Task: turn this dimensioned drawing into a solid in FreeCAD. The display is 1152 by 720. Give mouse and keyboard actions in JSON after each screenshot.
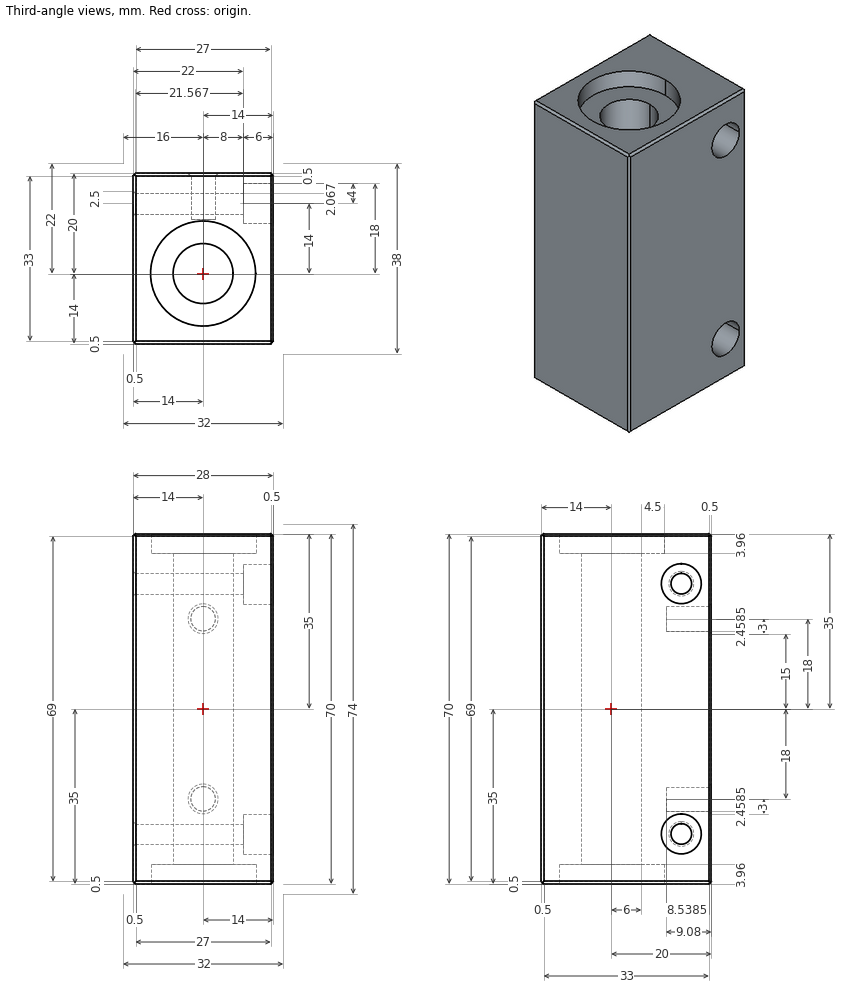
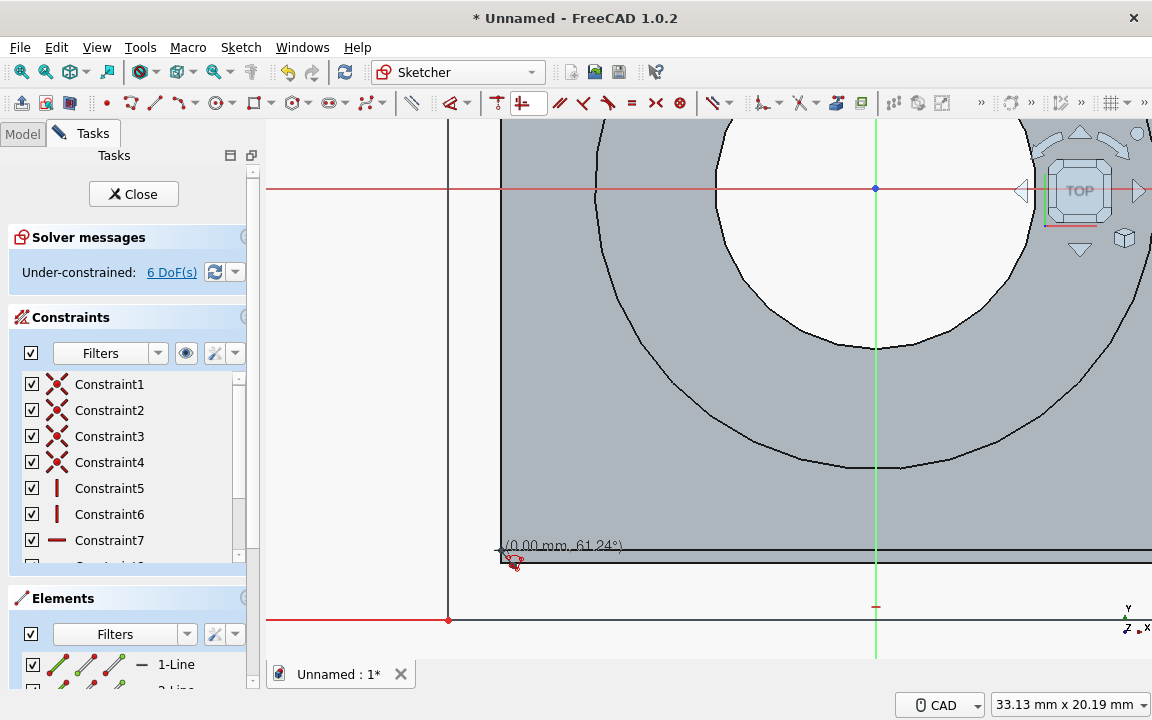
{"action": "scroll", "coordinate": [504, 552], "scroll_direction": "down", "scroll_amount": 5}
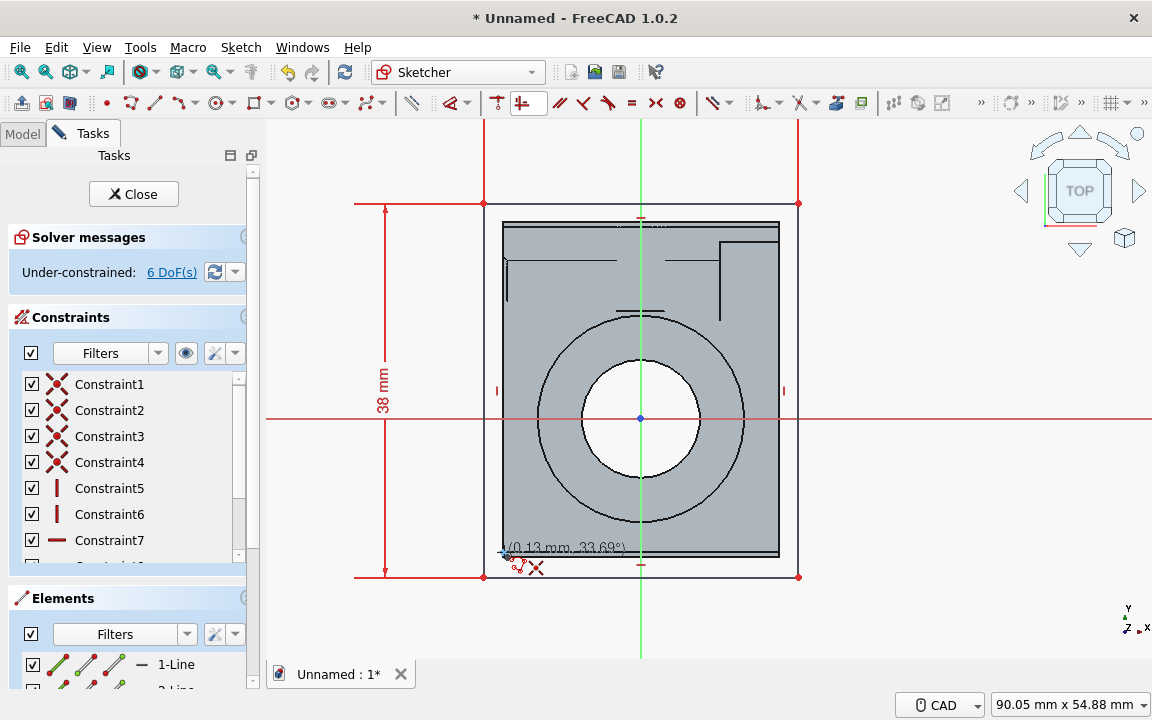
{"action": "left_click", "coordinate": [503, 227]}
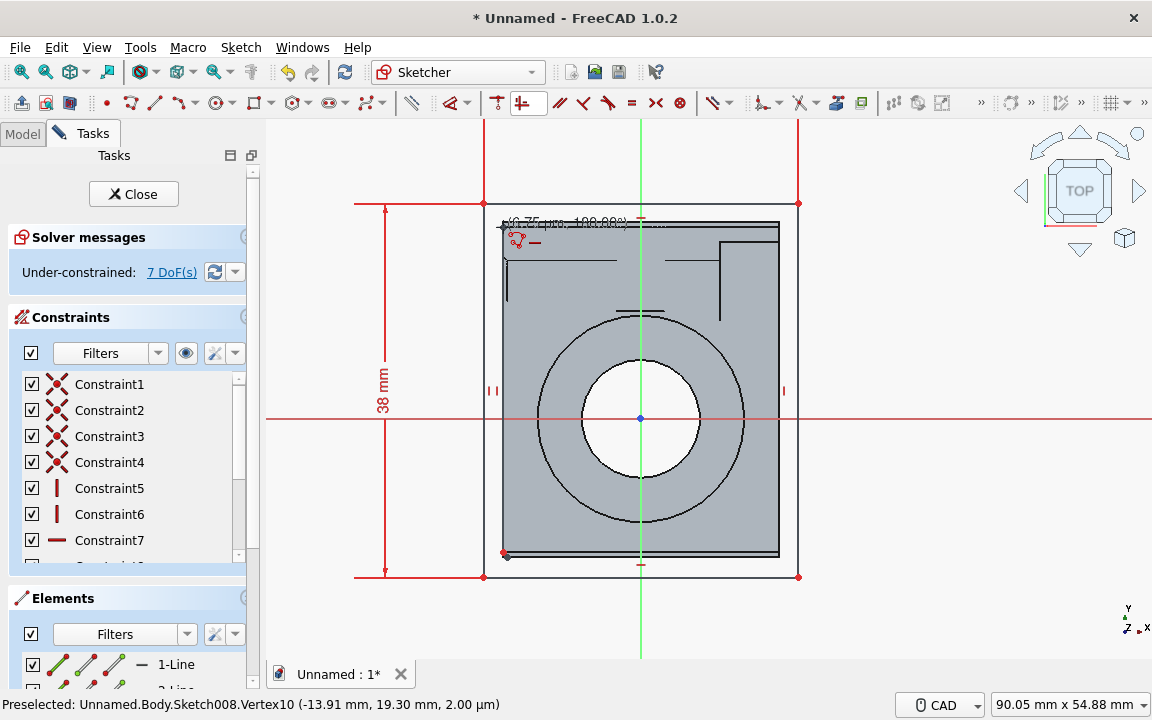
{"action": "scroll", "coordinate": [508, 222], "scroll_direction": "up", "scroll_amount": 5}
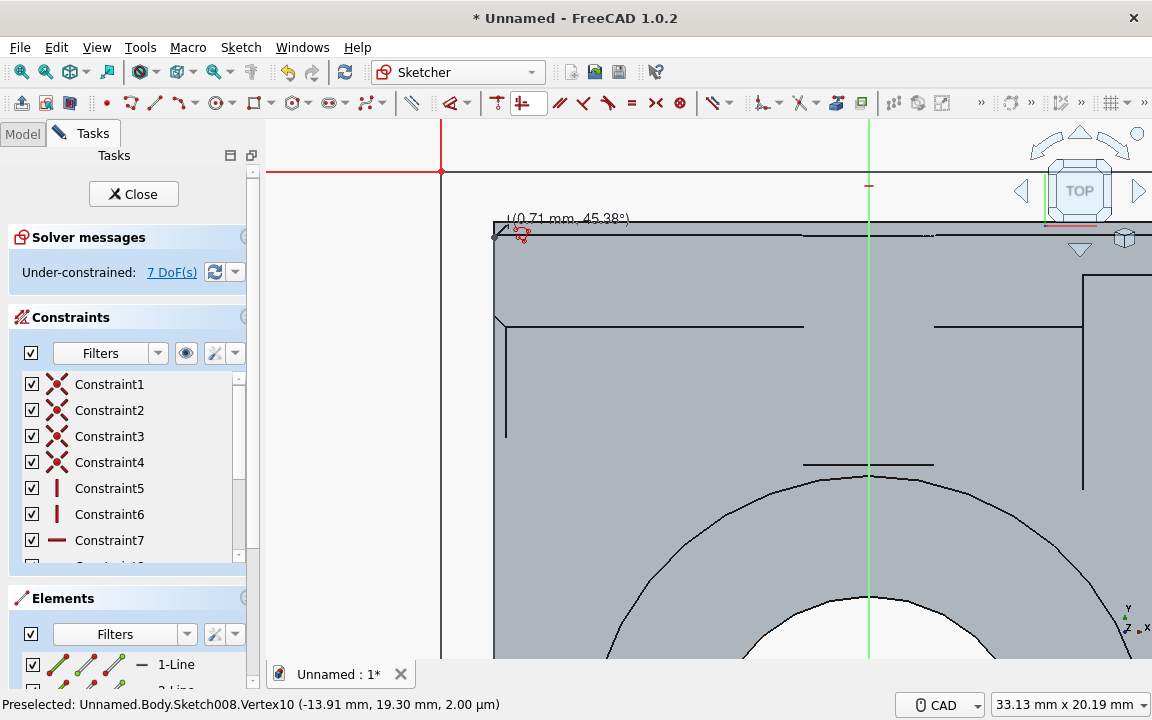
{"action": "left_click", "coordinate": [508, 222]}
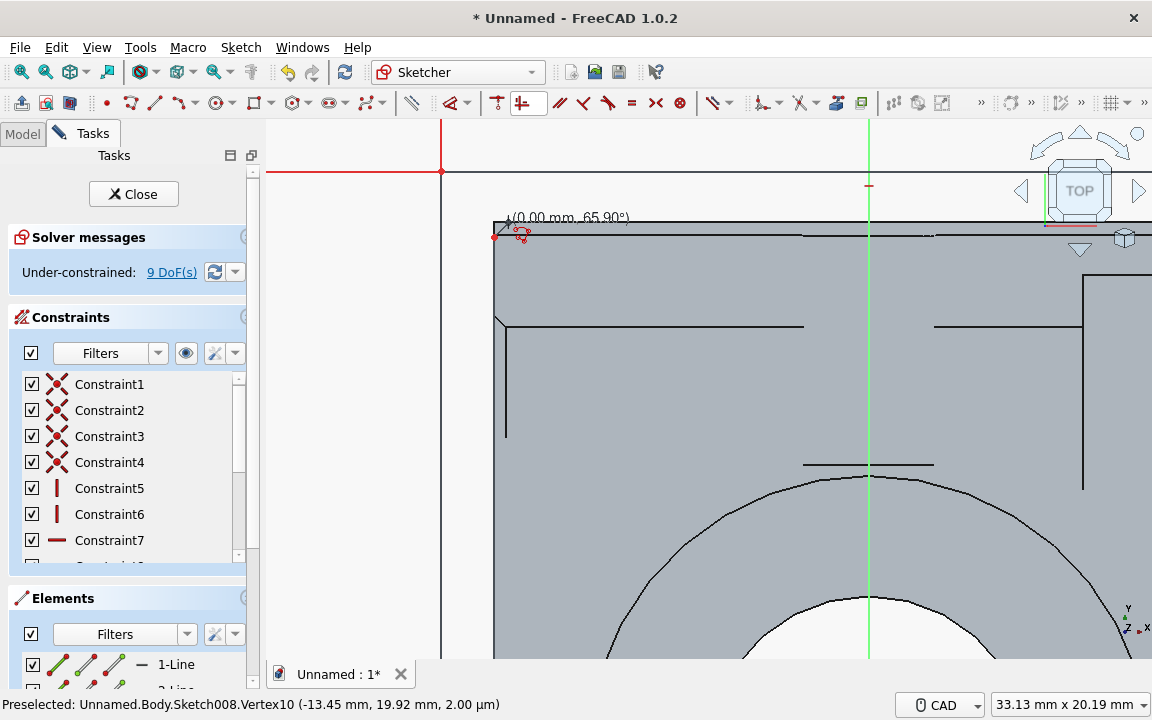
{"action": "scroll", "coordinate": [508, 222], "scroll_direction": "down", "scroll_amount": 5}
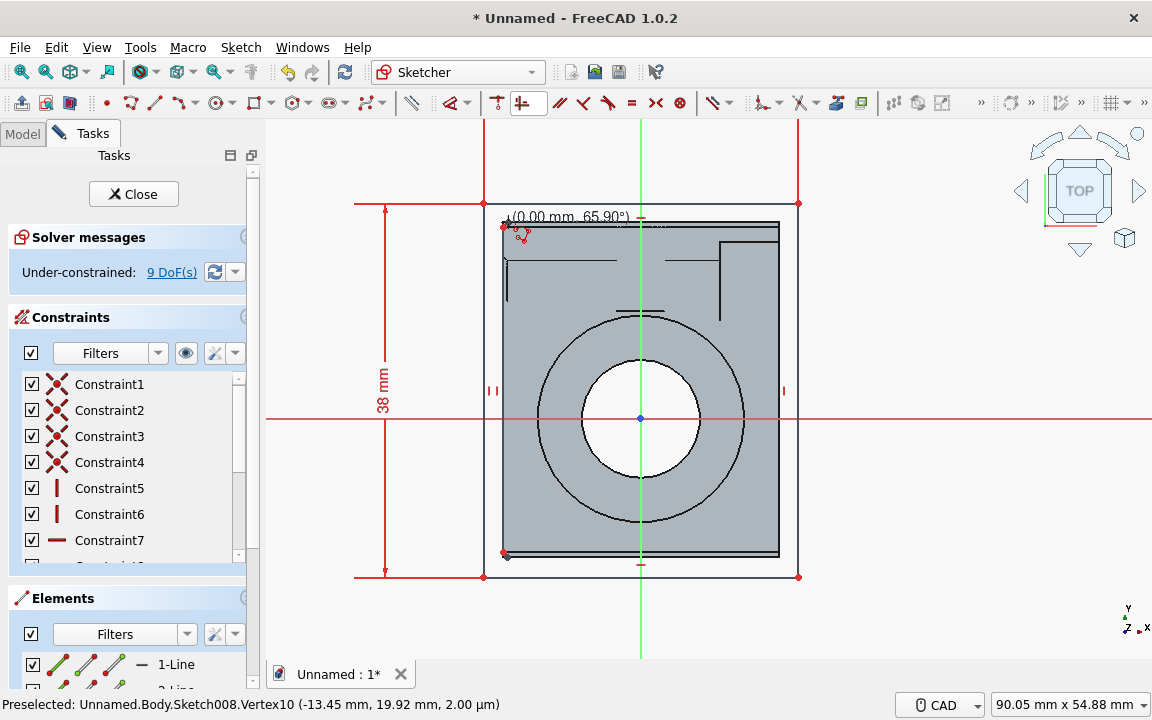
{"action": "left_click", "coordinate": [774, 222]}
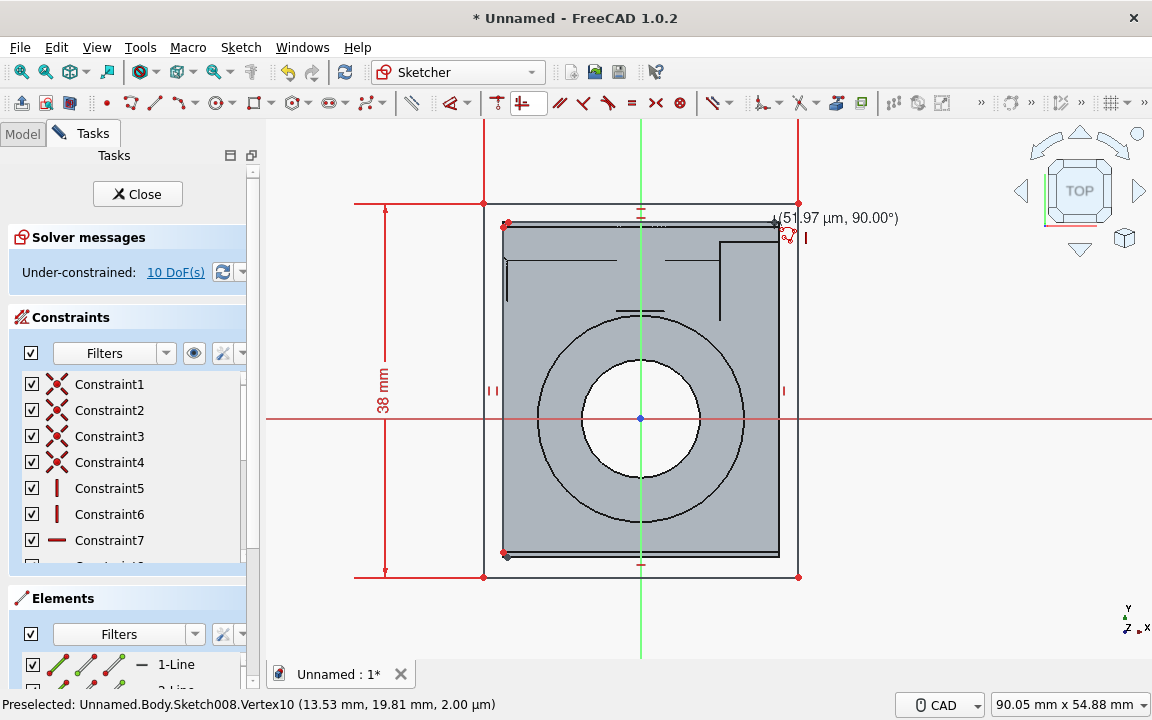
{"action": "scroll", "coordinate": [779, 227], "scroll_direction": "up", "scroll_amount": 5}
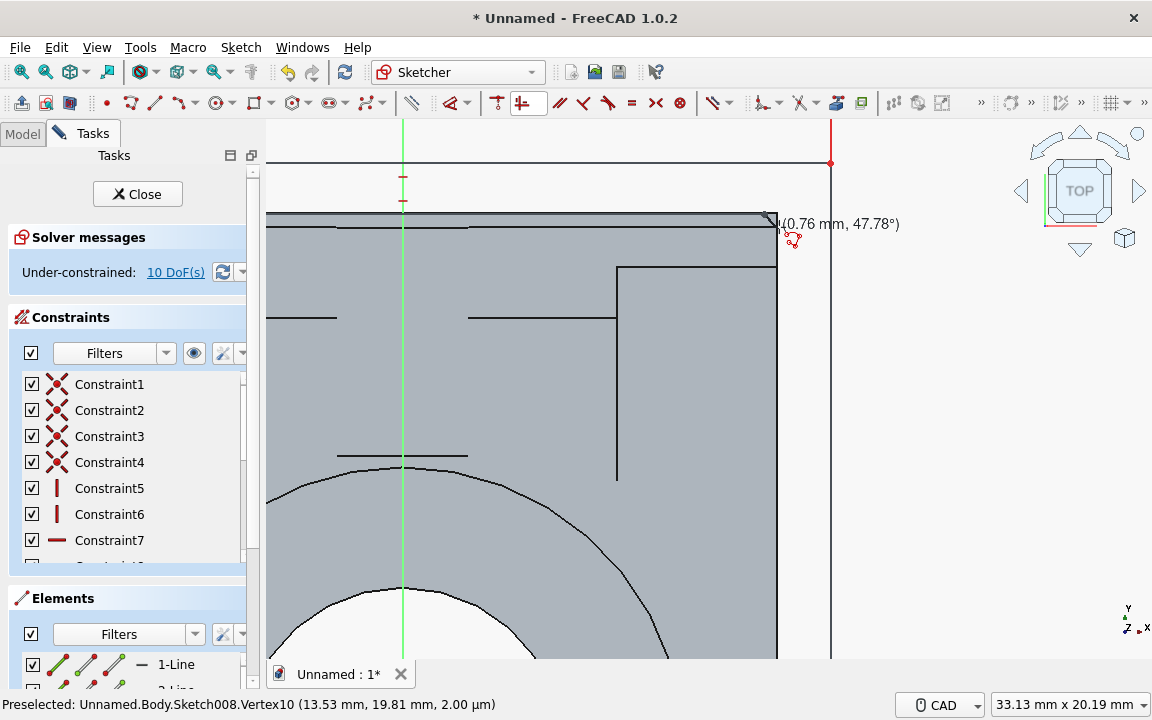
{"action": "left_click", "coordinate": [777, 227]}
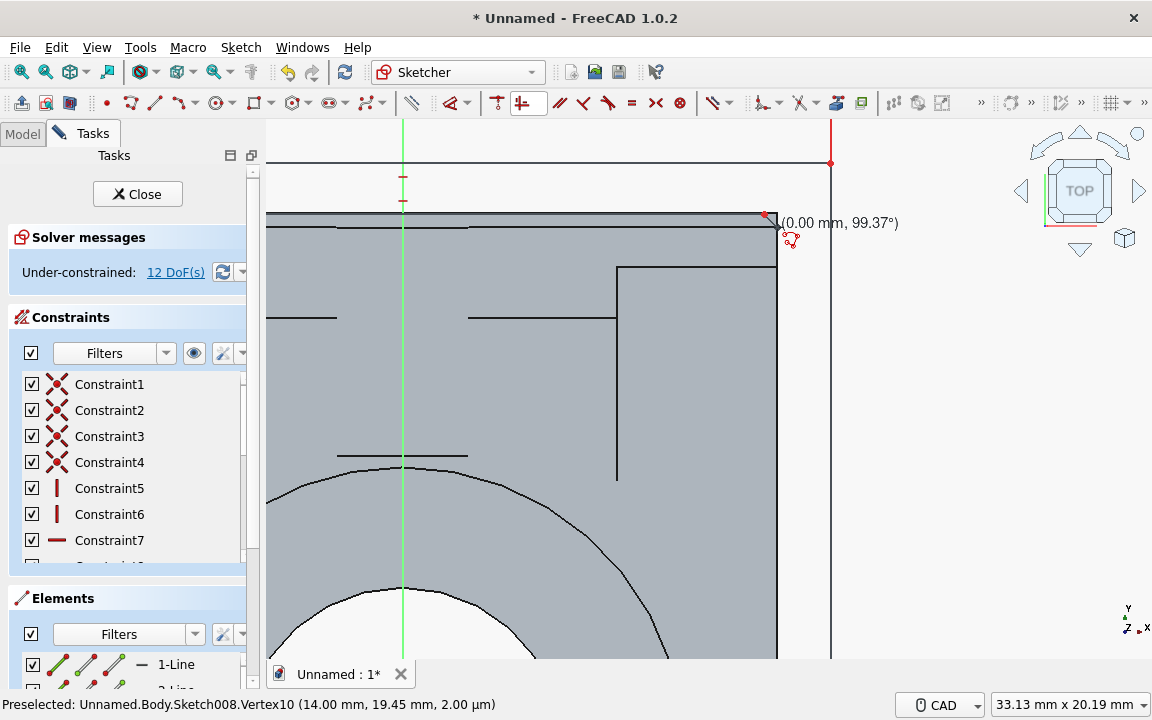
{"action": "scroll", "coordinate": [779, 227], "scroll_direction": "down", "scroll_amount": 5}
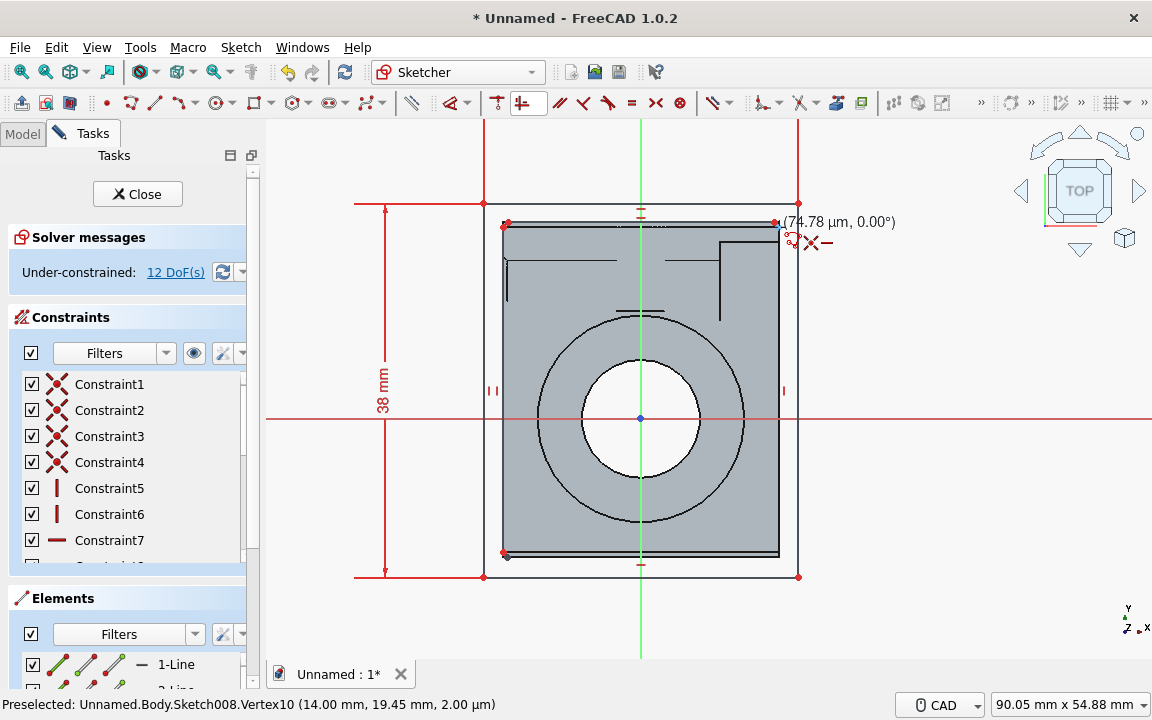
{"action": "left_click", "coordinate": [779, 552]}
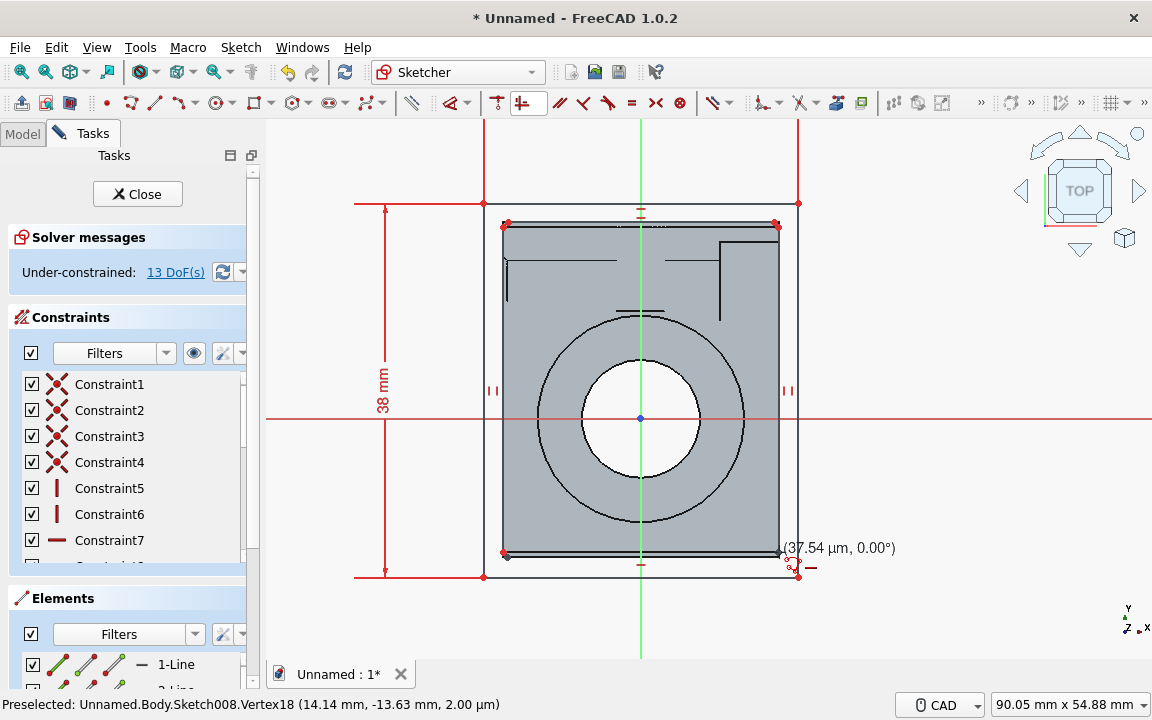
{"action": "scroll", "coordinate": [774, 557], "scroll_direction": "up", "scroll_amount": 5}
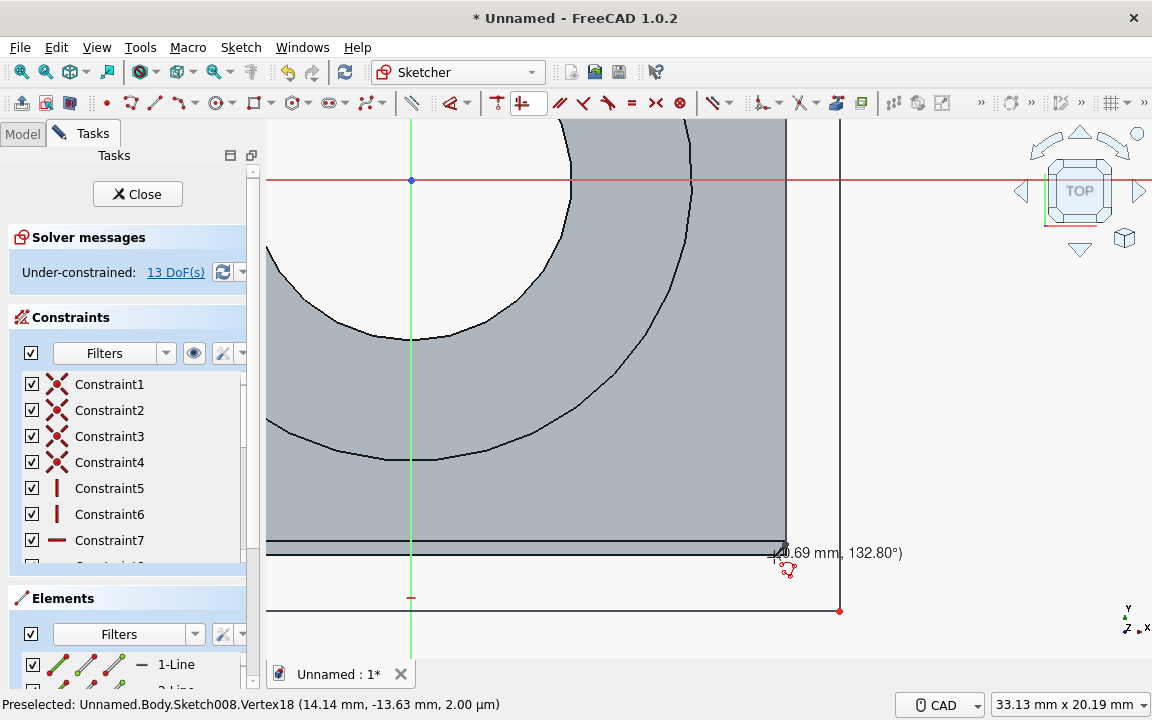
{"action": "left_click", "coordinate": [772, 555]}